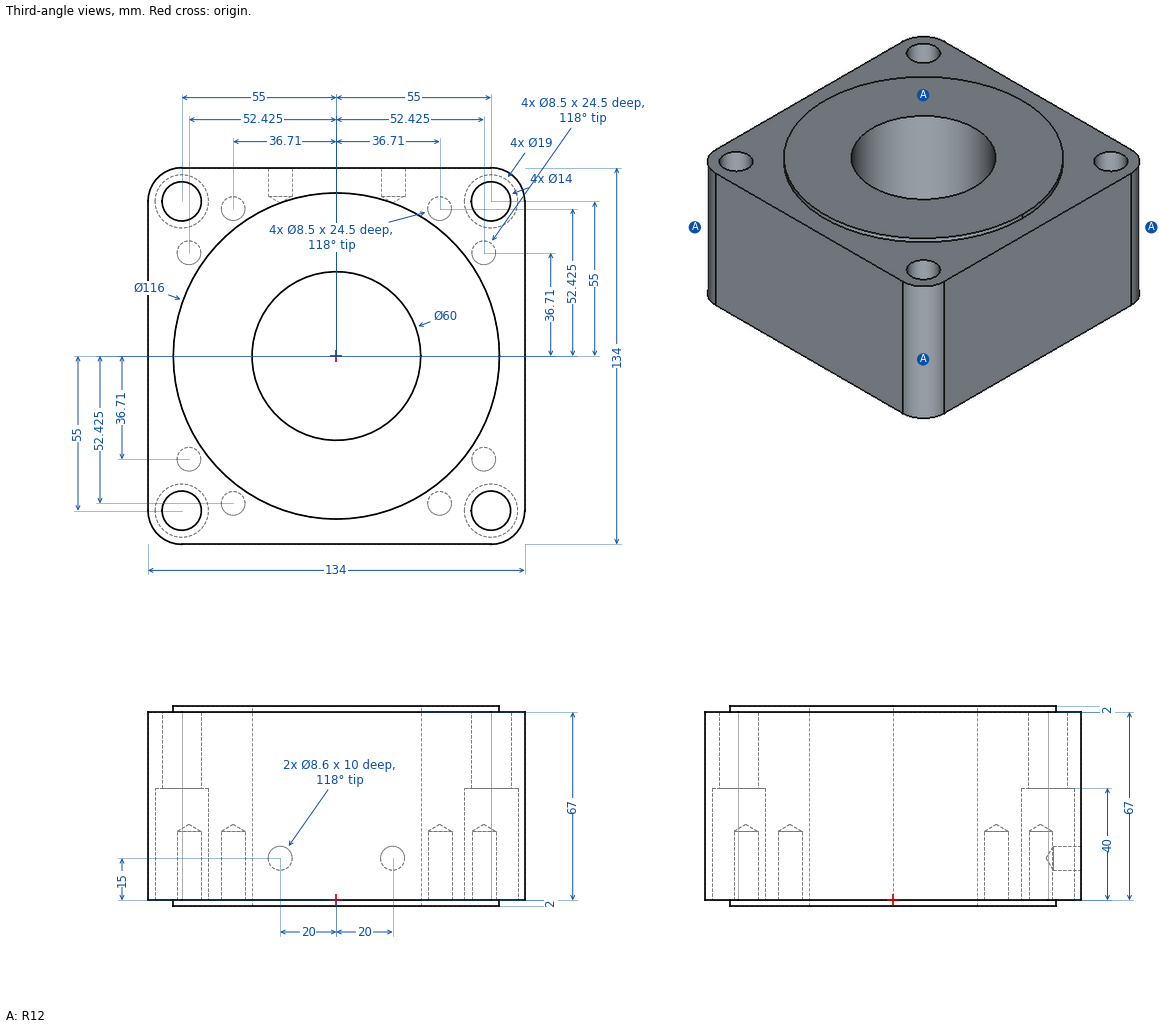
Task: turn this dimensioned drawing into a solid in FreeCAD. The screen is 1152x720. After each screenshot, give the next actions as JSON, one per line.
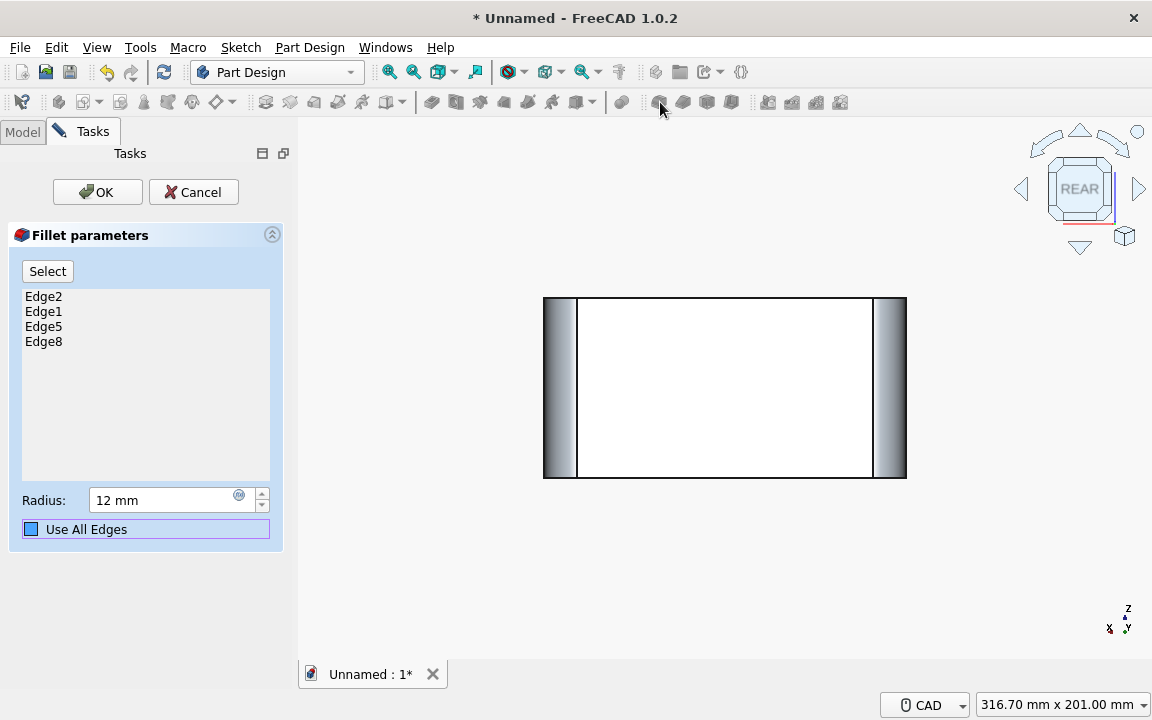
{"action": "left_click", "coordinate": [98, 192]}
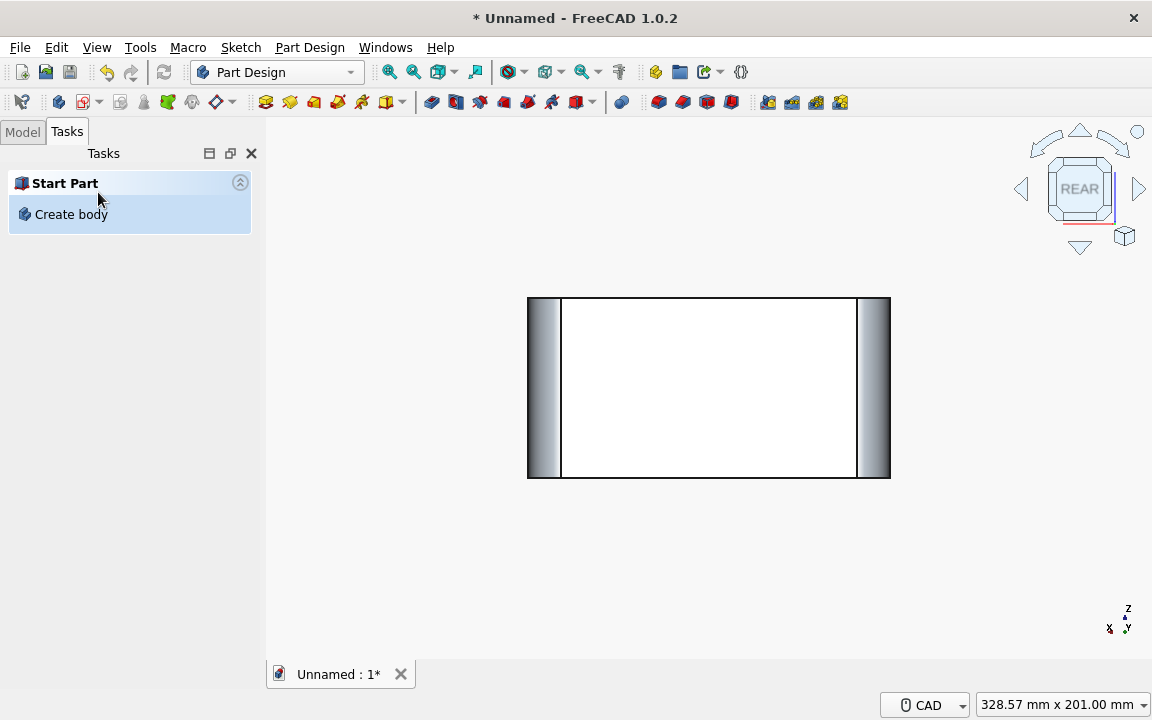
{"action": "left_click", "coordinate": [390, 72]}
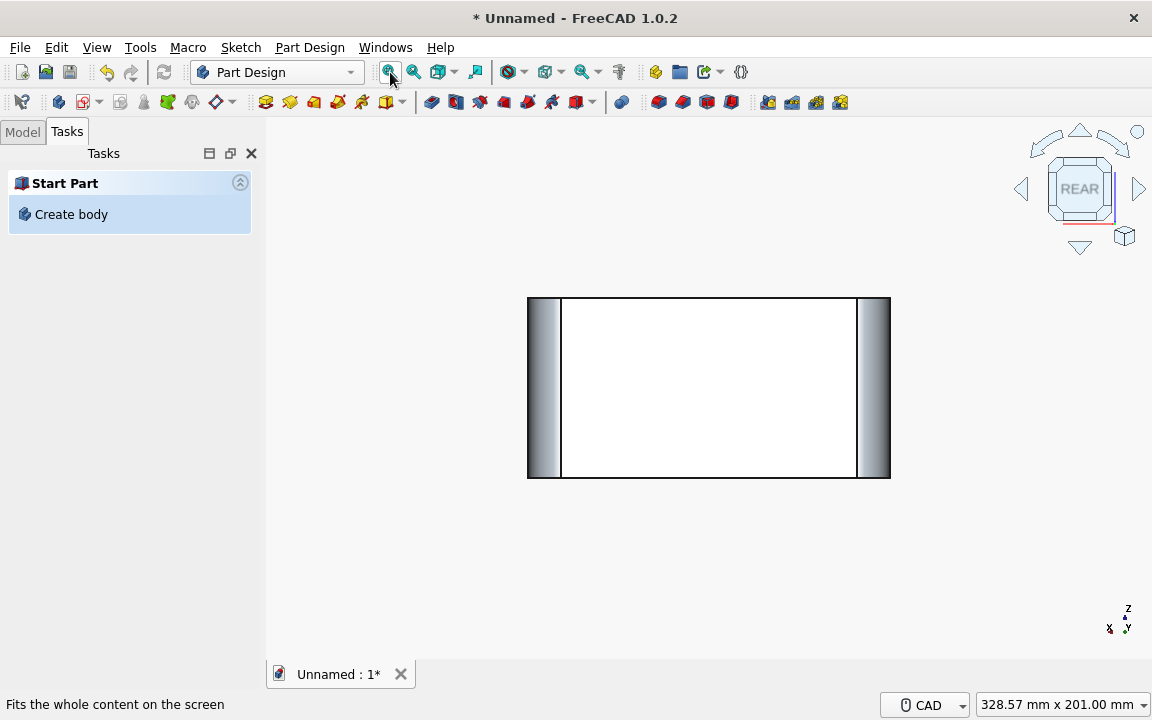
{"action": "key", "text": "0"}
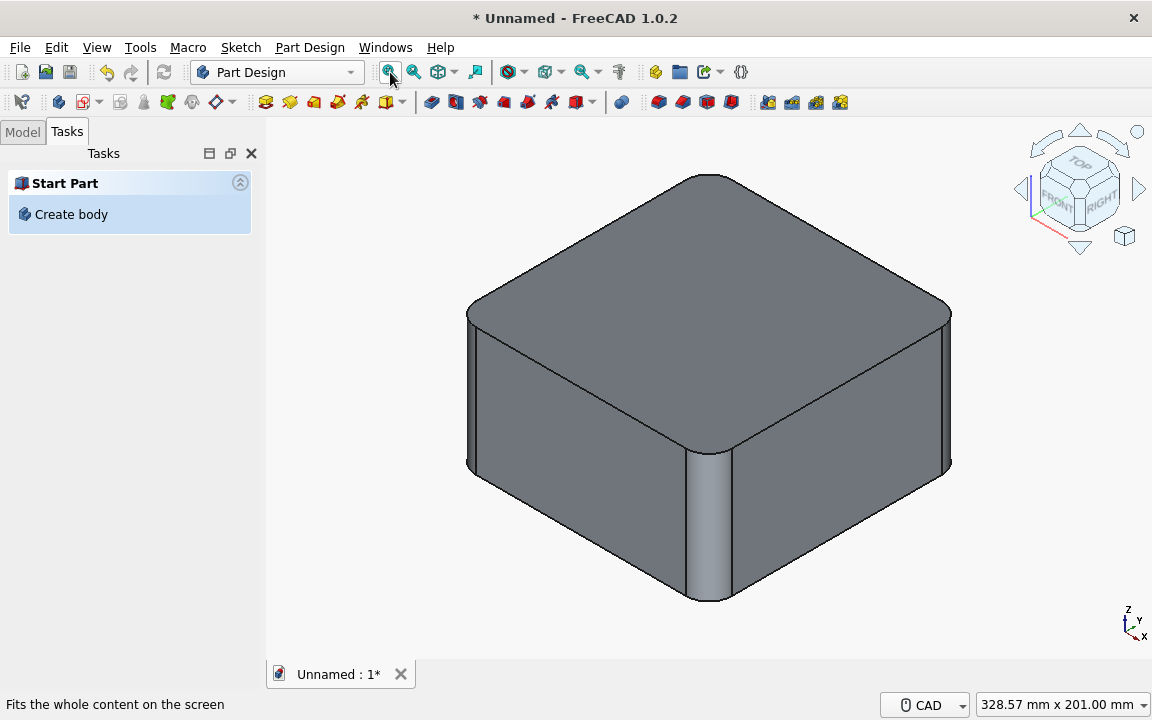
{"action": "left_click", "coordinate": [709, 313]}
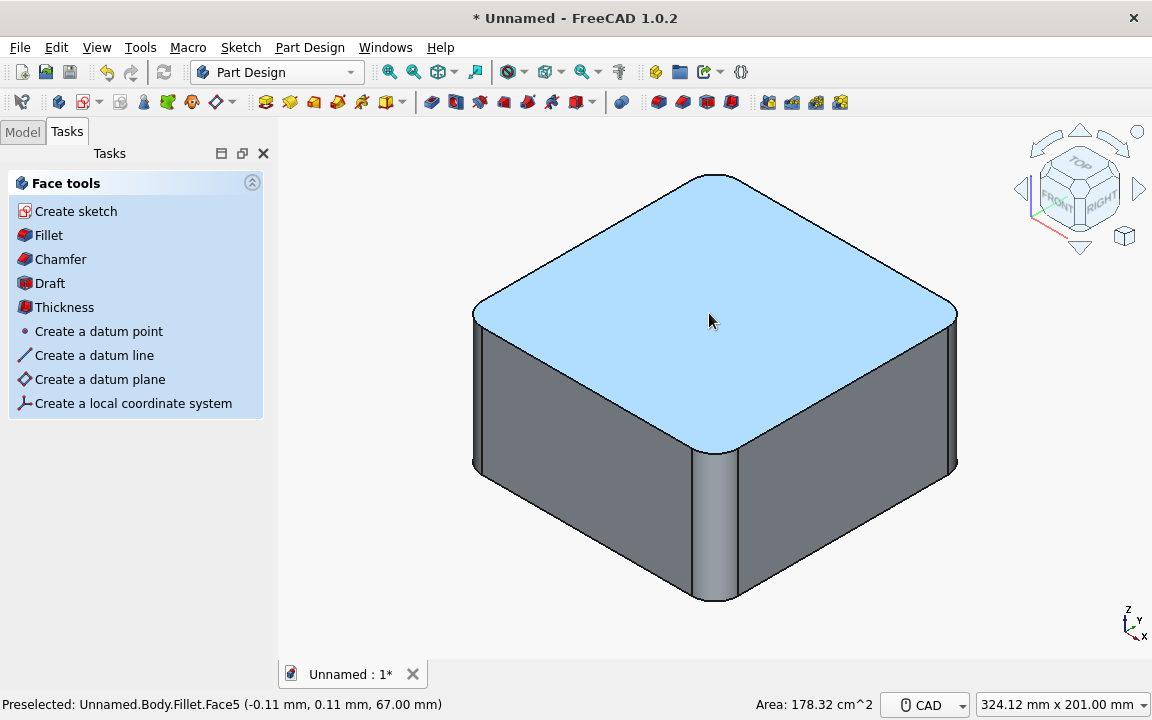
{"action": "left_click", "coordinate": [84, 102]}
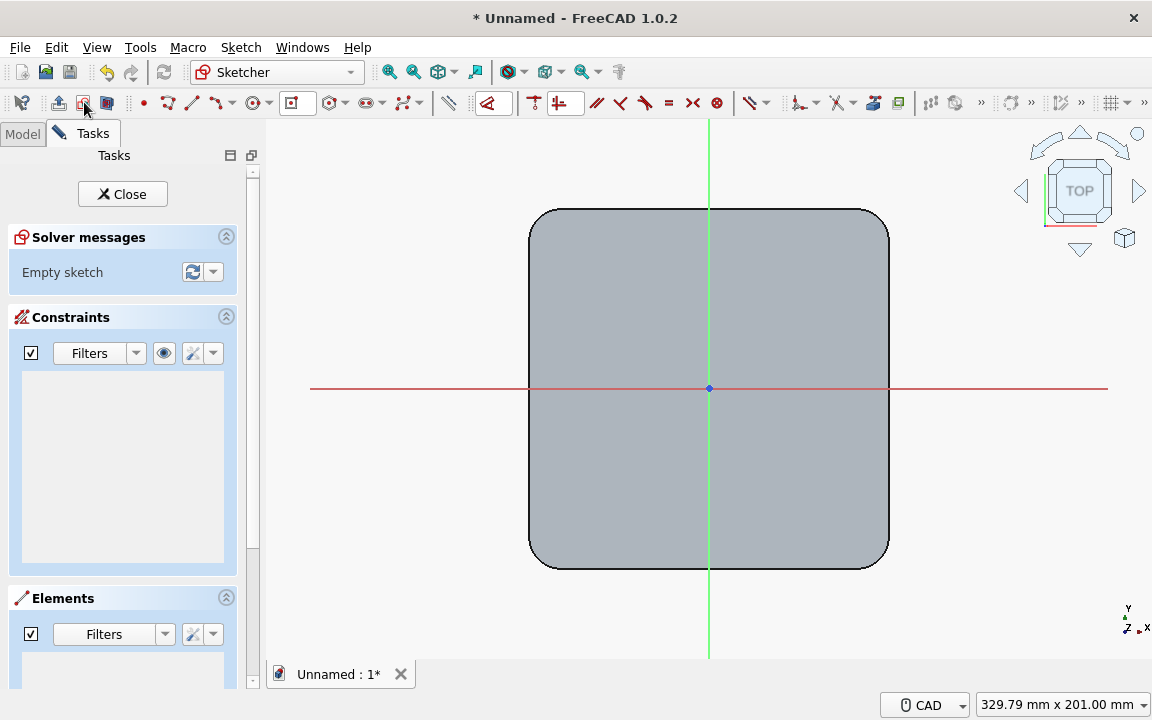
{"action": "scroll", "coordinate": [765, 389], "scroll_direction": "up", "scroll_amount": 4}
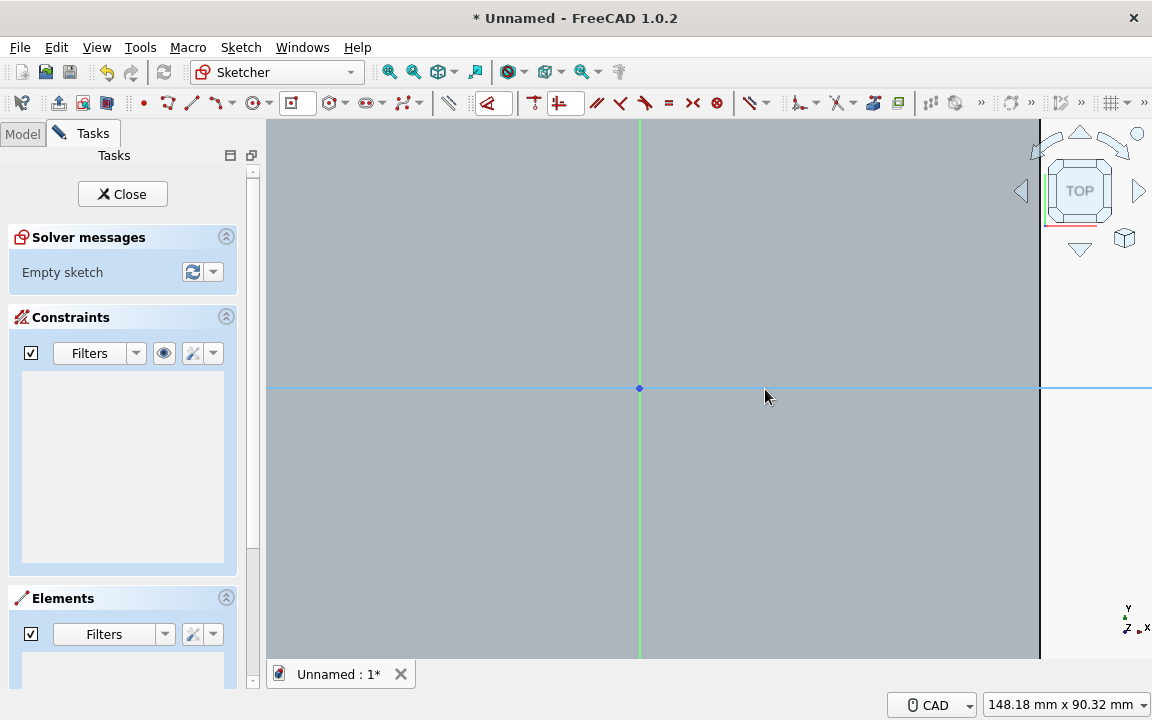
{"action": "left_click", "coordinate": [254, 104]}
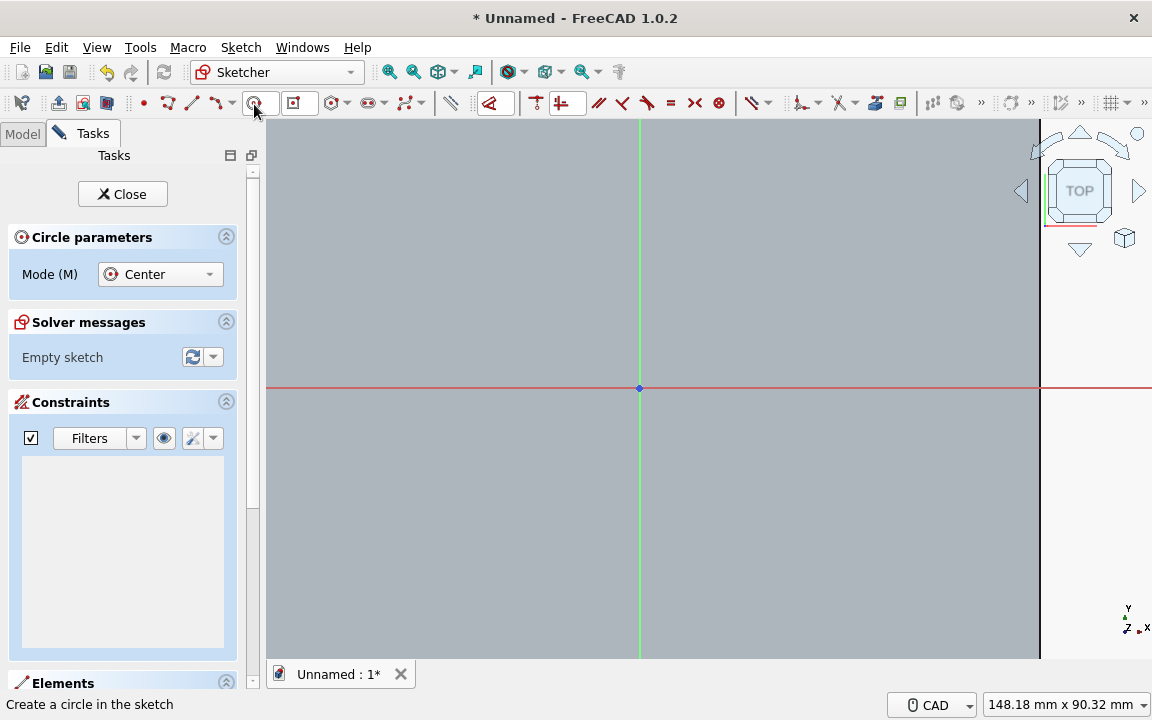
{"action": "left_click", "coordinate": [640, 388]}
{"action": "left_click", "coordinate": [767, 262]}
{"action": "key", "text": "Escape"}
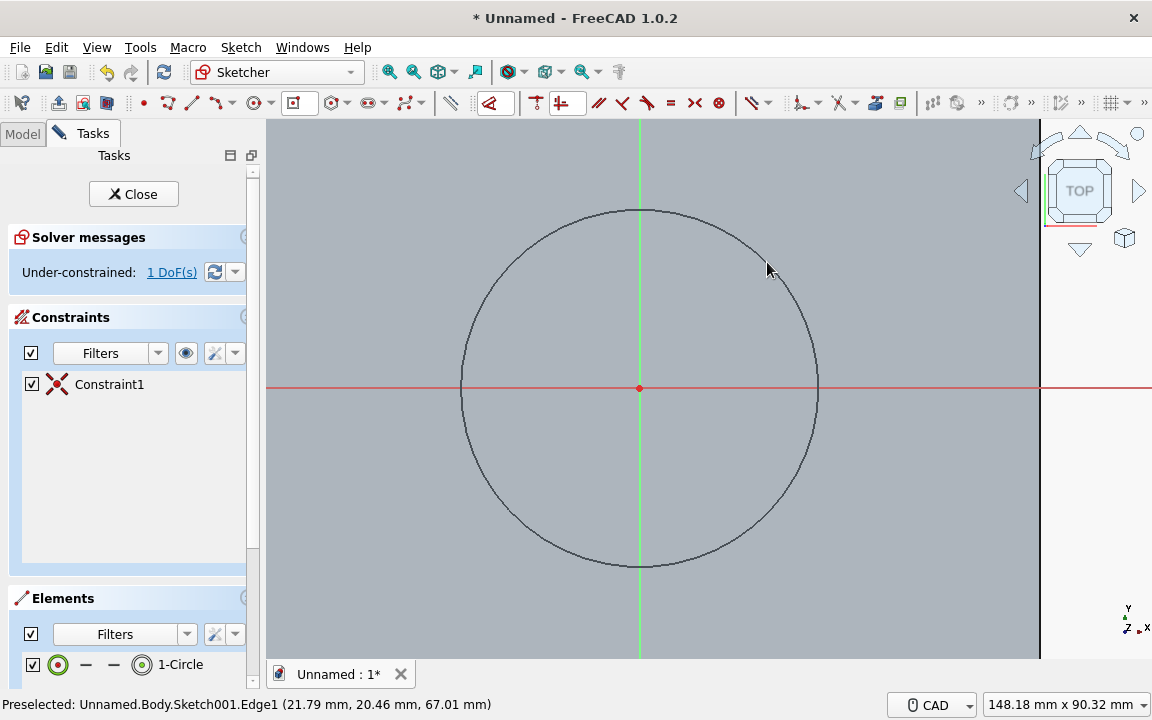
{"action": "left_click", "coordinate": [766, 262]}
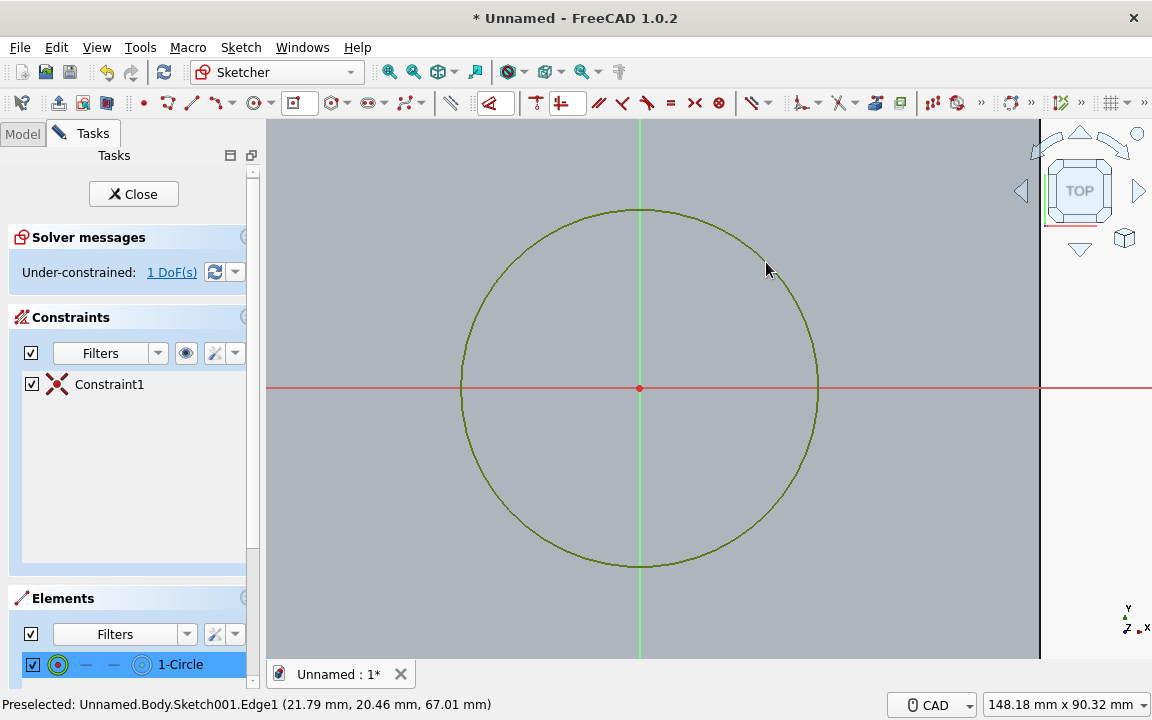
{"action": "key", "text": "k o"}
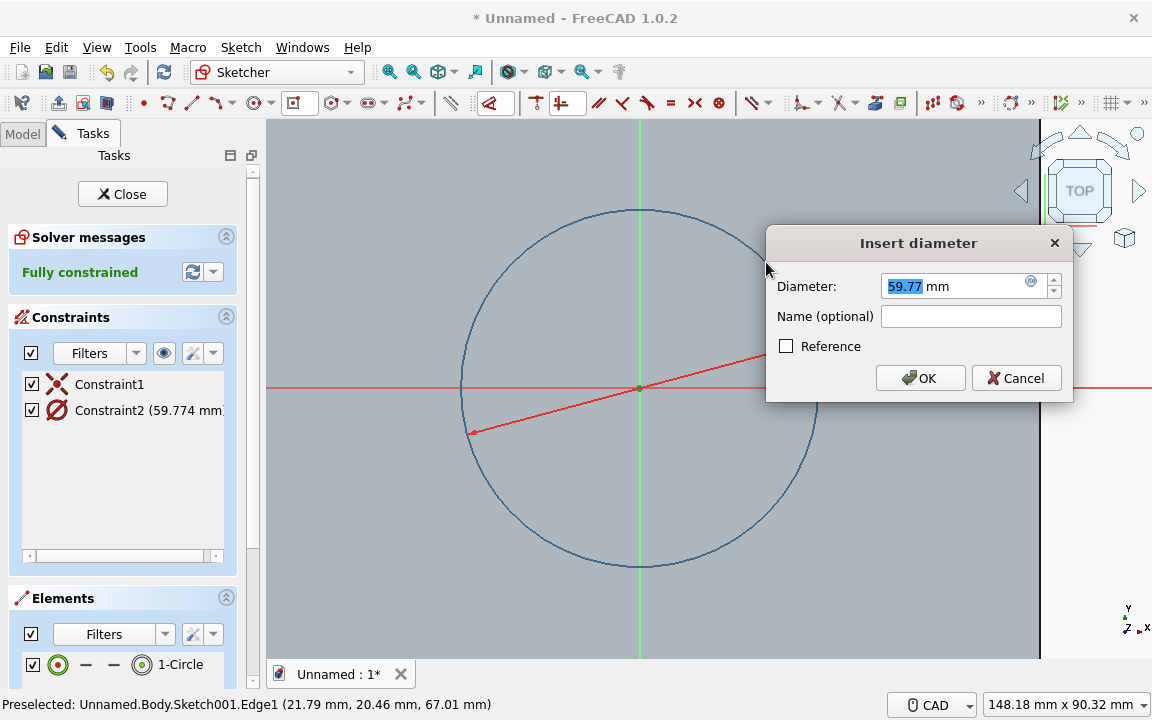
{"action": "type", "text": "60"}
{"action": "key", "text": "Return"}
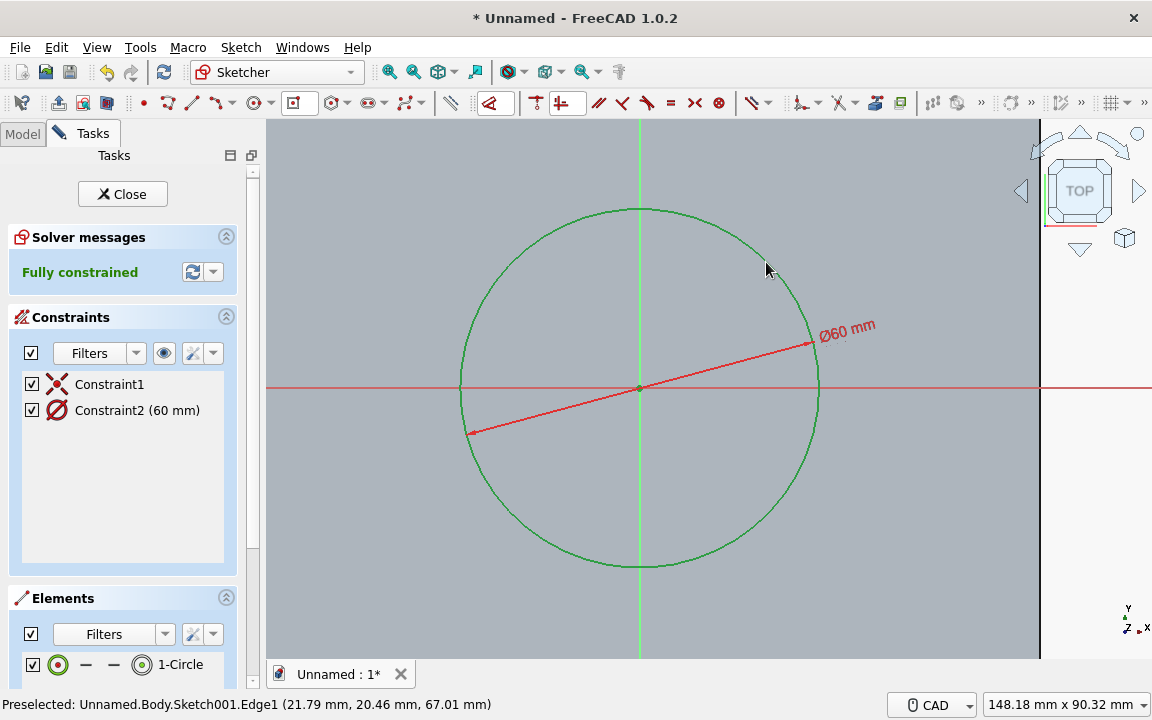
{"action": "left_click", "coordinate": [123, 194]}